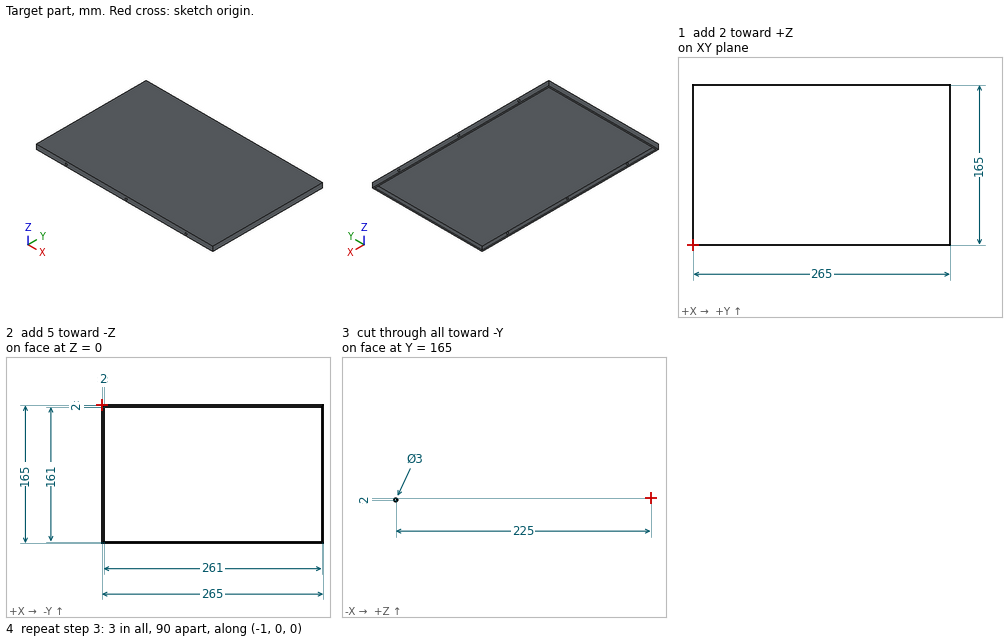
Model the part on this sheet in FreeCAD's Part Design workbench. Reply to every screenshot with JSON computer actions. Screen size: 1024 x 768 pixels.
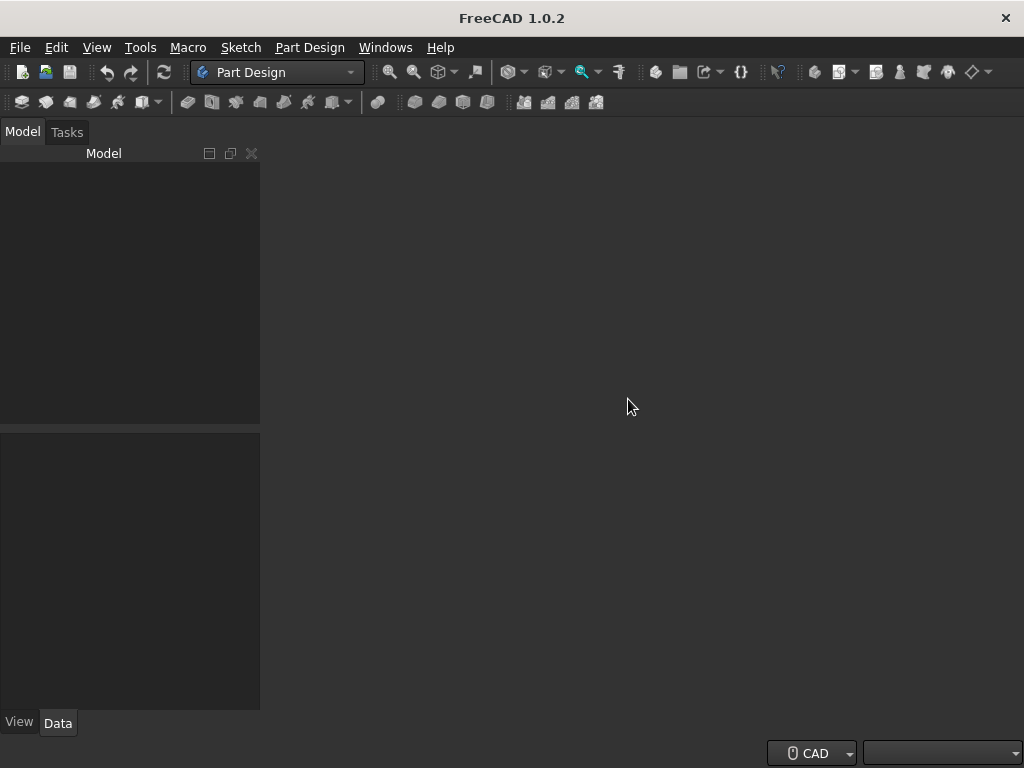
{"action": "key", "text": "ctrl+n"}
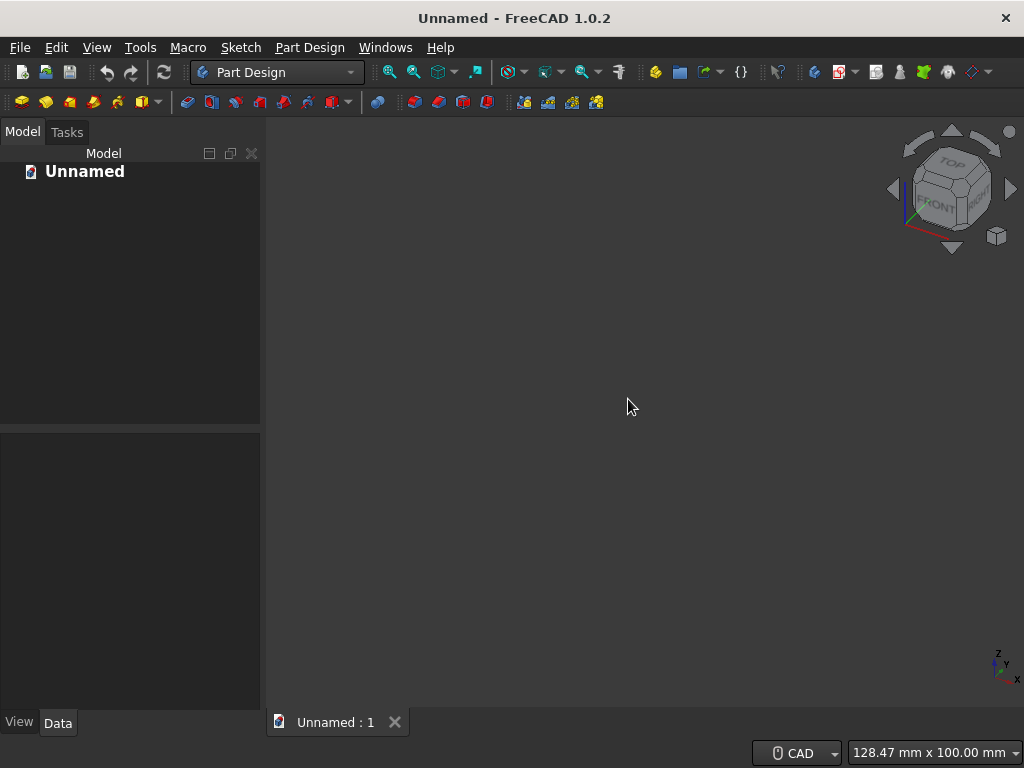
{"action": "left_click", "coordinate": [840, 72]}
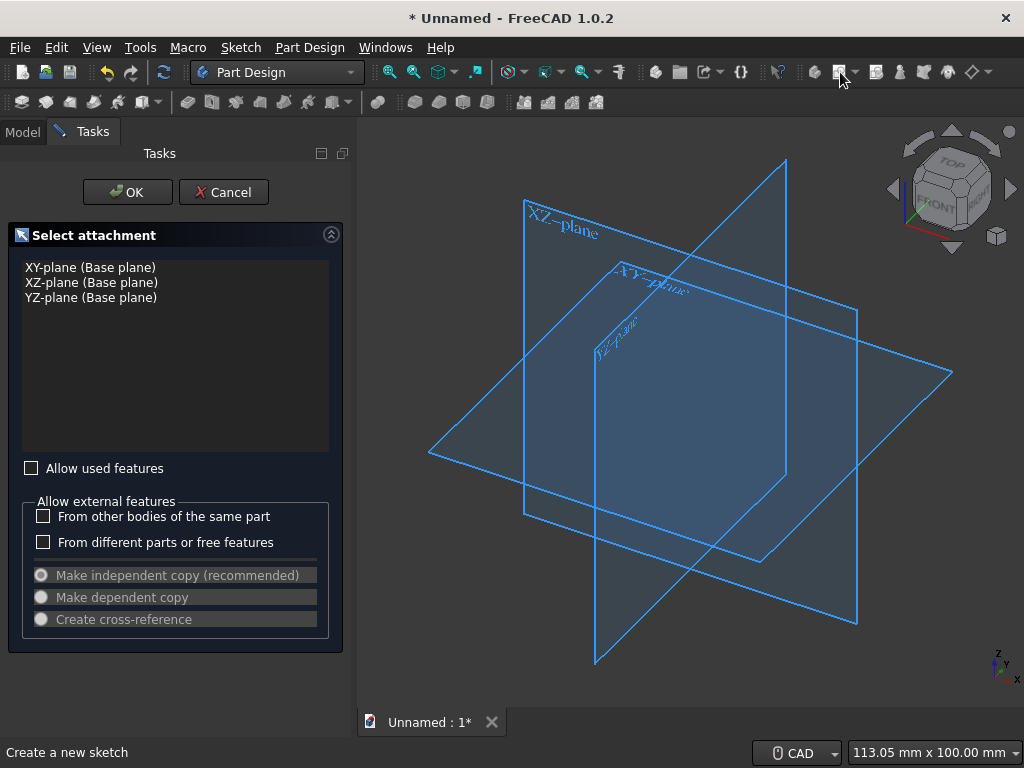
{"action": "left_click", "coordinate": [82, 268]}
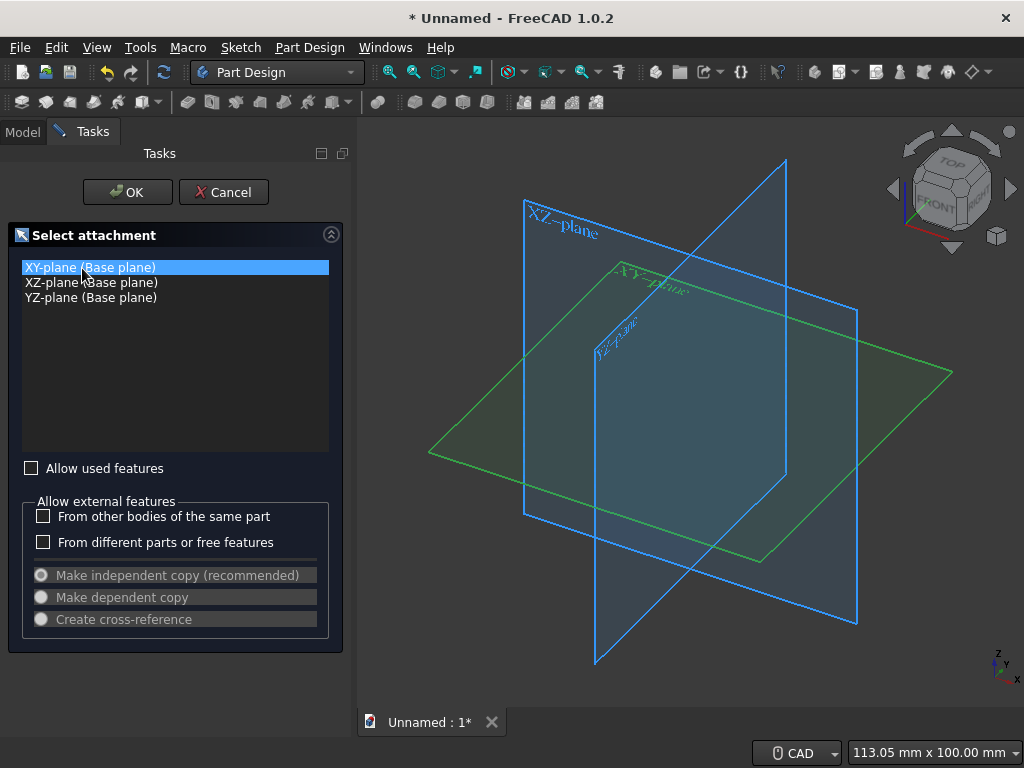
{"action": "left_click", "coordinate": [128, 192]}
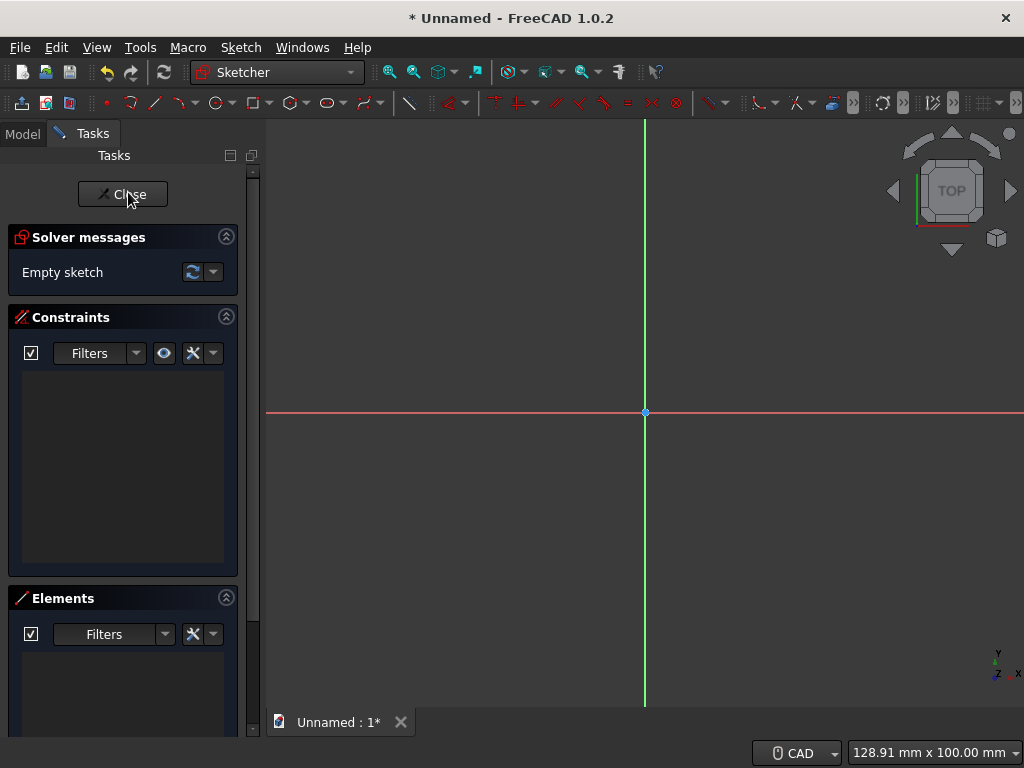
{"action": "scroll", "coordinate": [299, 572], "scroll_direction": "down", "scroll_amount": 7}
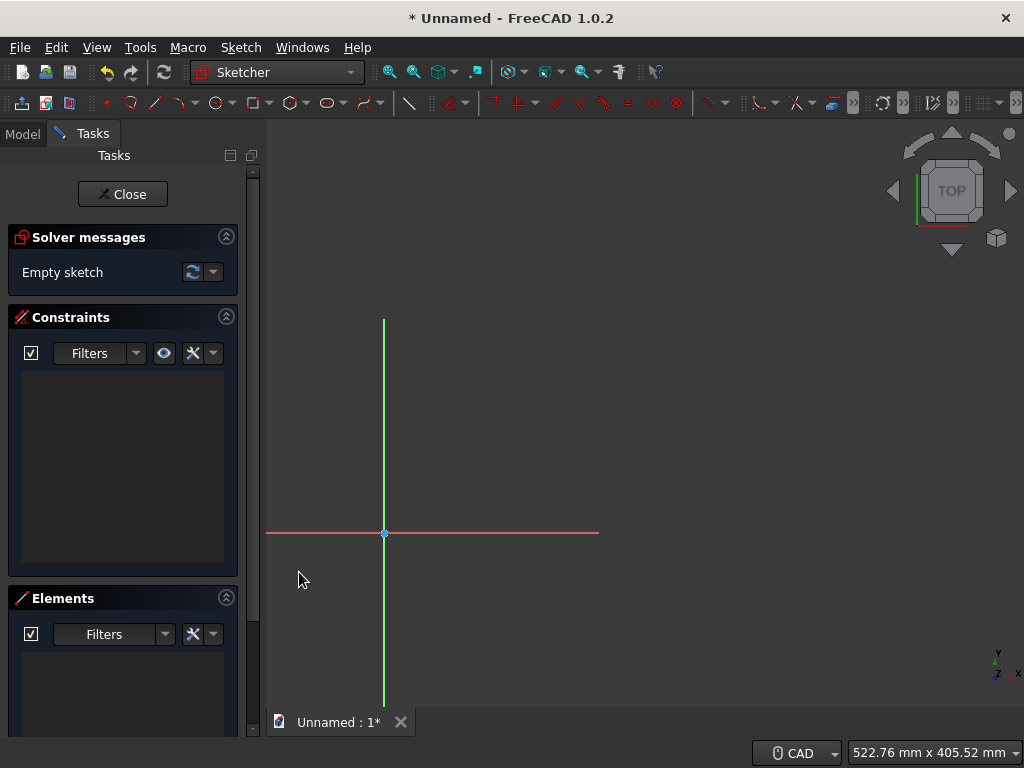
{"action": "key", "text": "g r"}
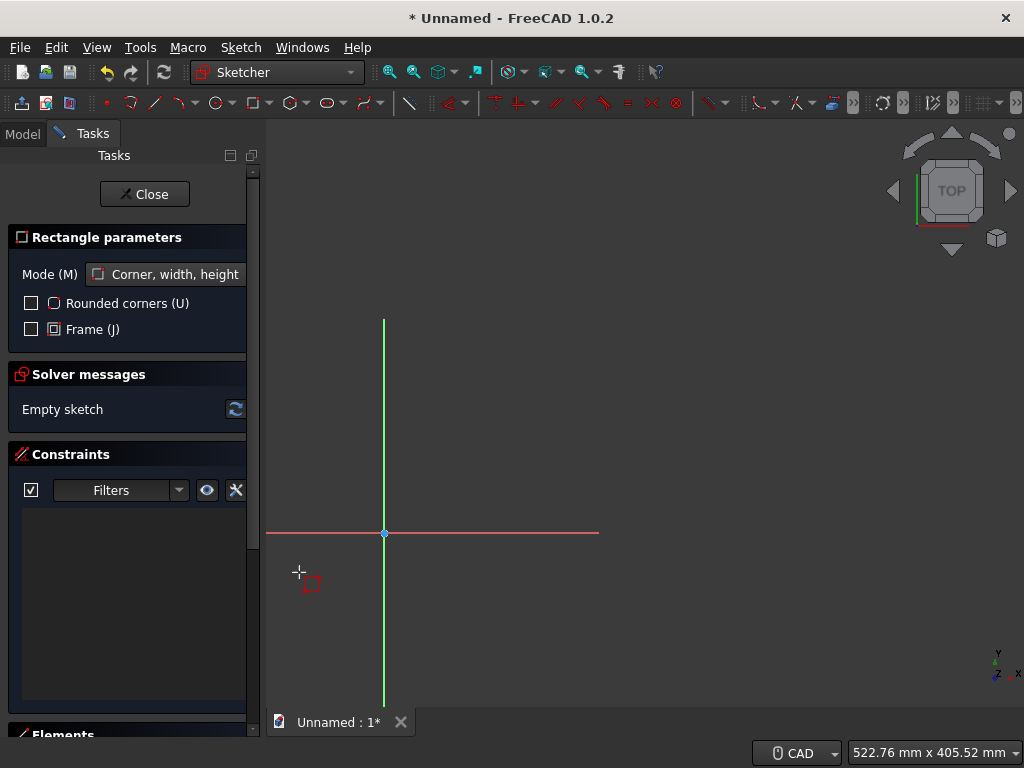
{"action": "left_click", "coordinate": [384, 533]}
{"action": "left_click", "coordinate": [769, 294]}
{"action": "key", "text": "Escape"}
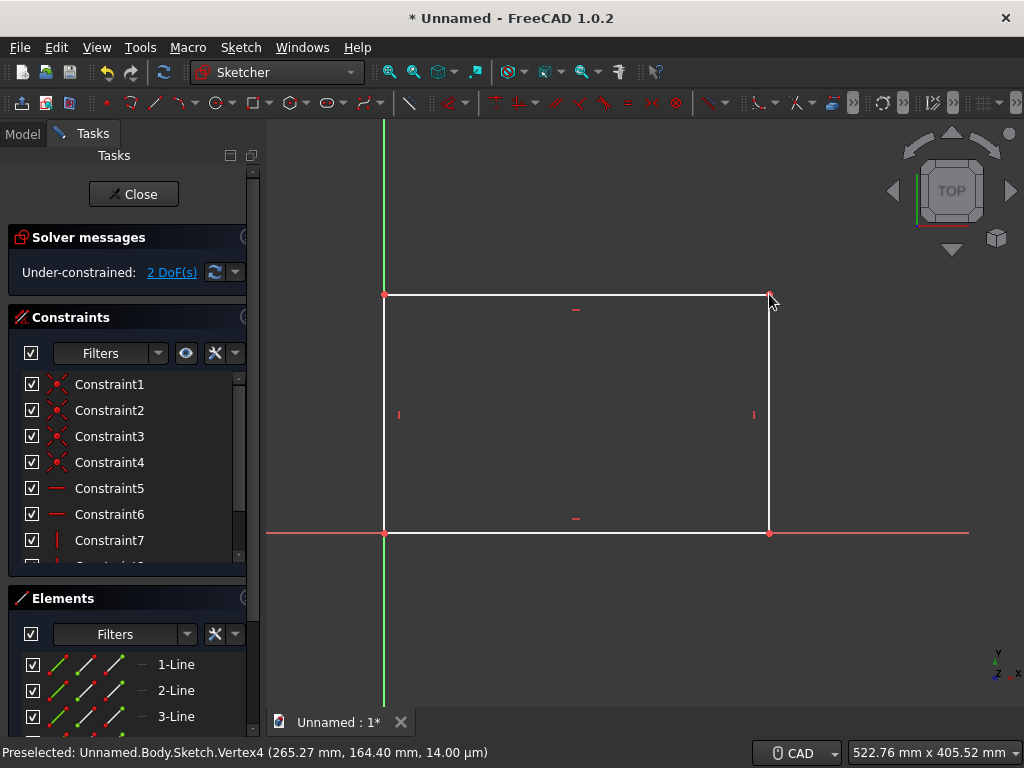
{"action": "left_click", "coordinate": [448, 104]}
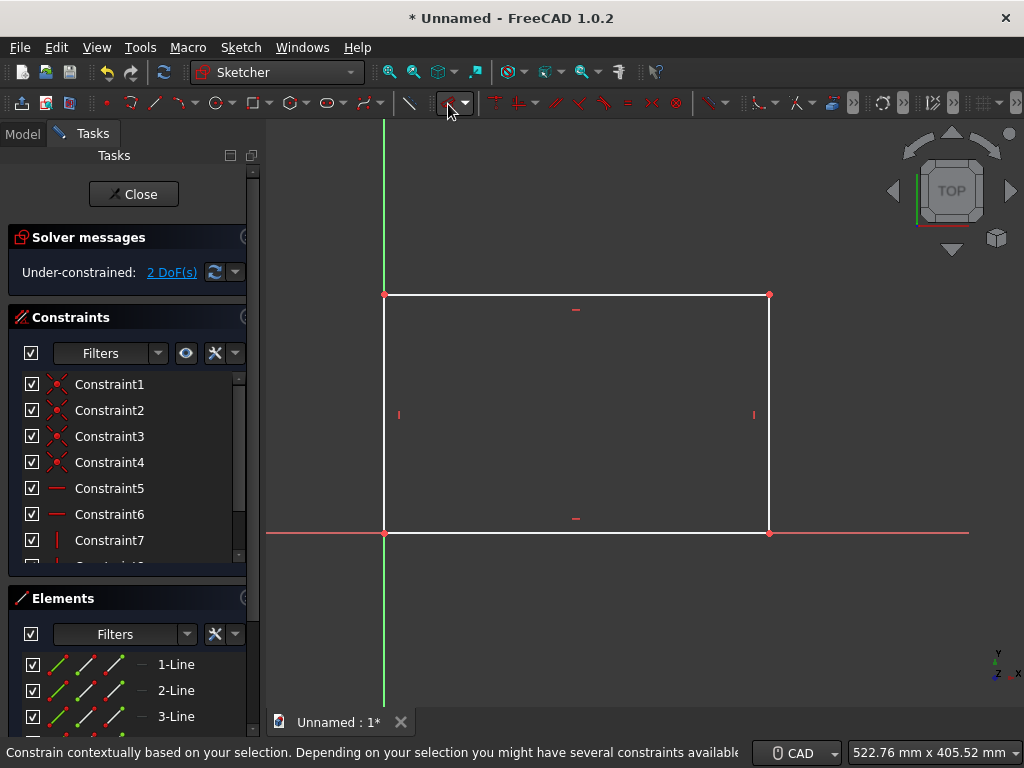
{"action": "left_click", "coordinate": [500, 533]}
{"action": "left_click", "coordinate": [577, 567]}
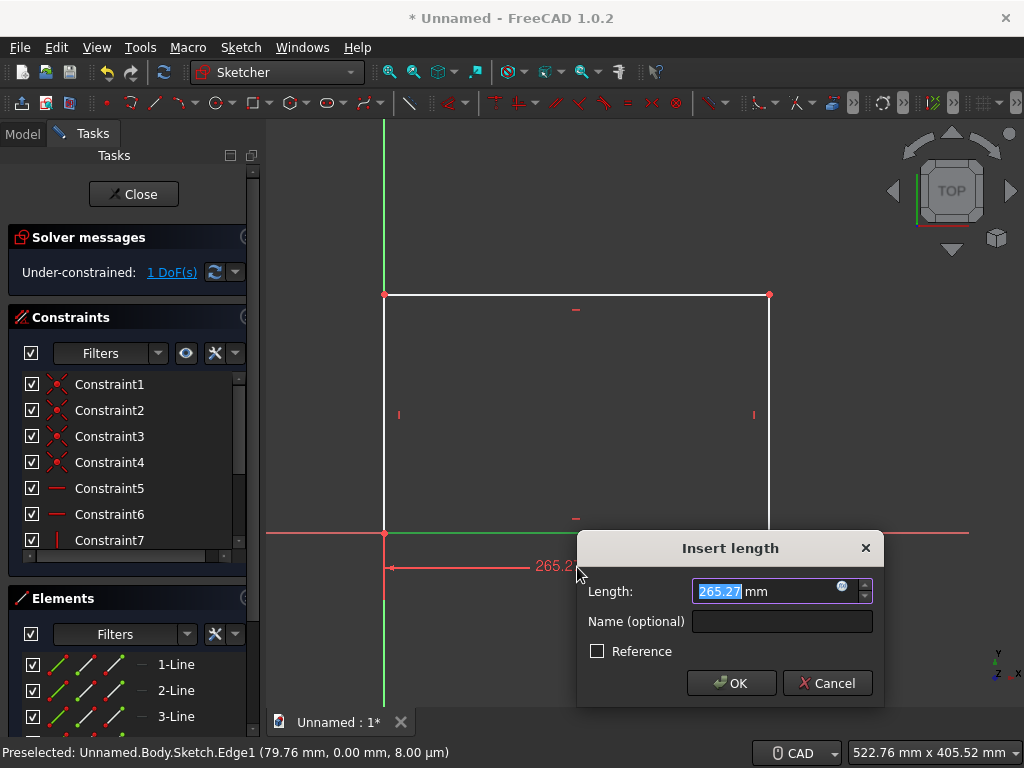
{"action": "type", "text": "265"}
{"action": "key", "text": "Return"}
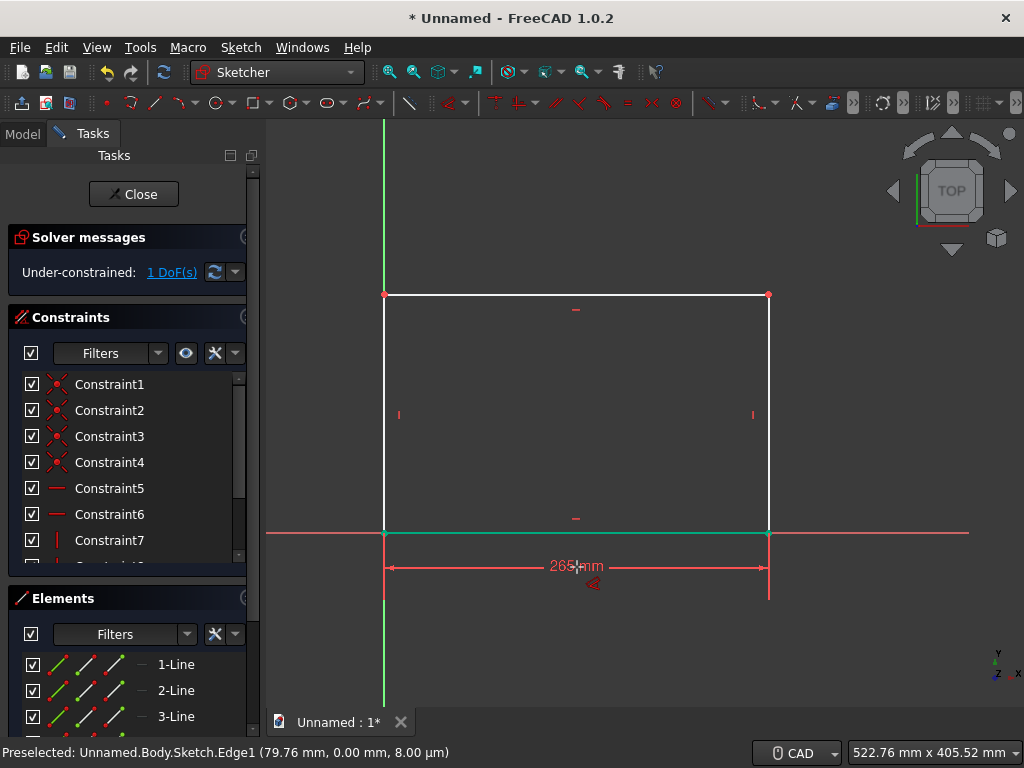
{"action": "left_click", "coordinate": [769, 462]}
{"action": "left_click", "coordinate": [803, 414]}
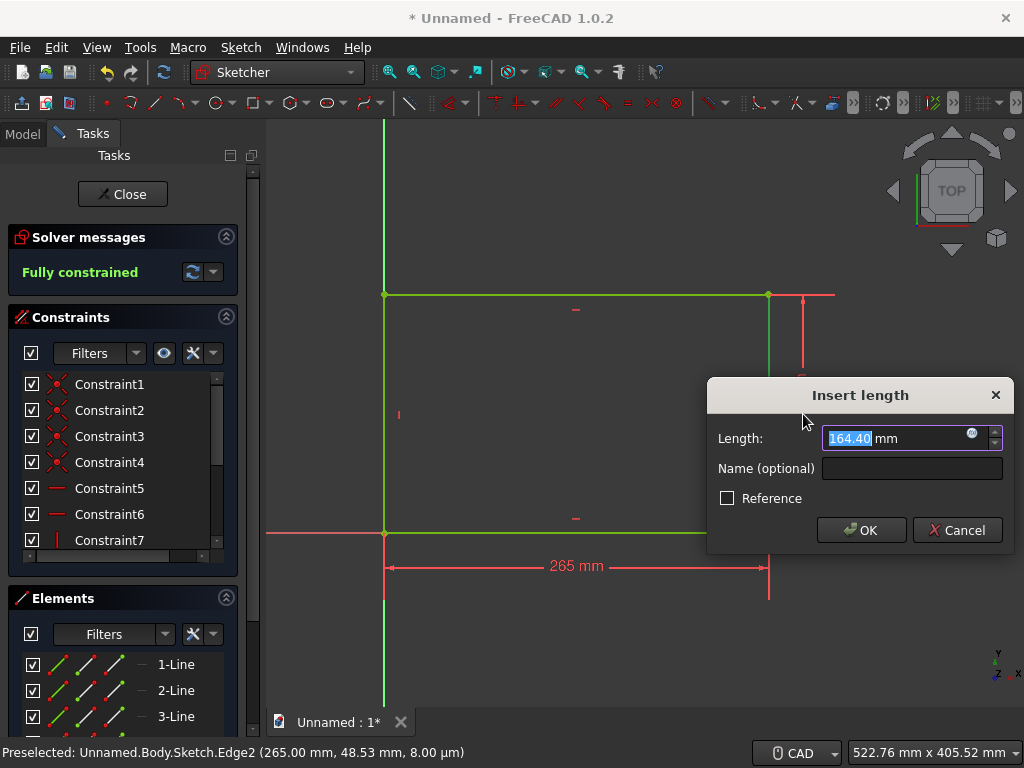
{"action": "type", "text": "165"}
{"action": "key", "text": "Return"}
{"action": "key", "text": "Escape"}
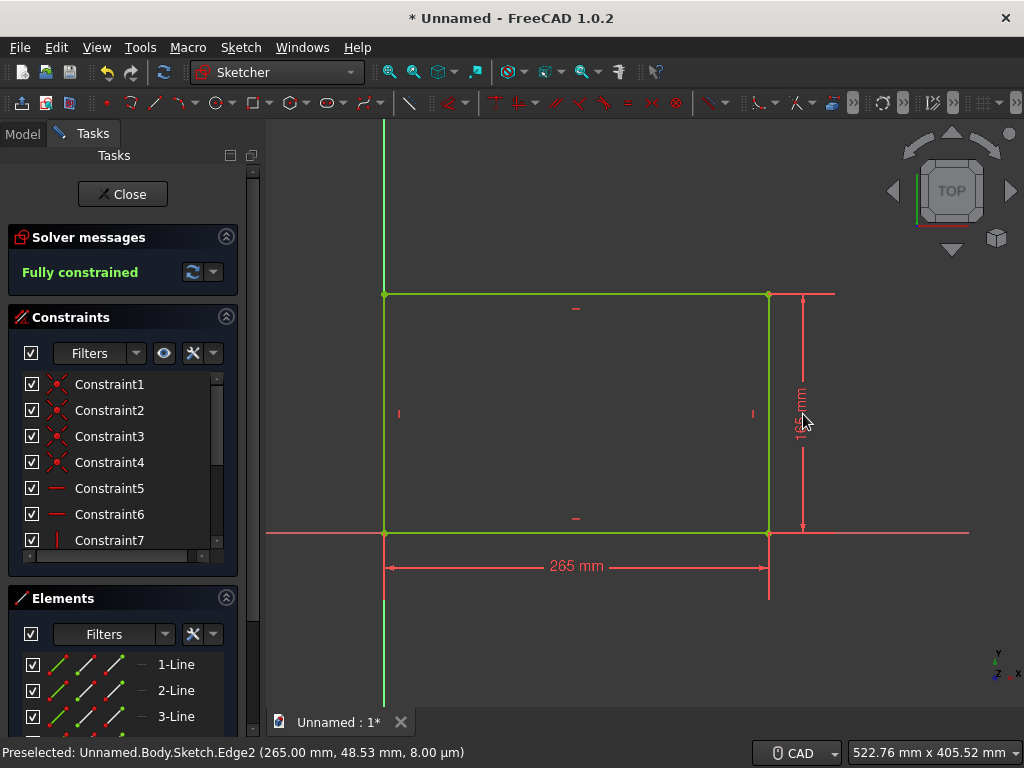
{"action": "left_click", "coordinate": [123, 194]}